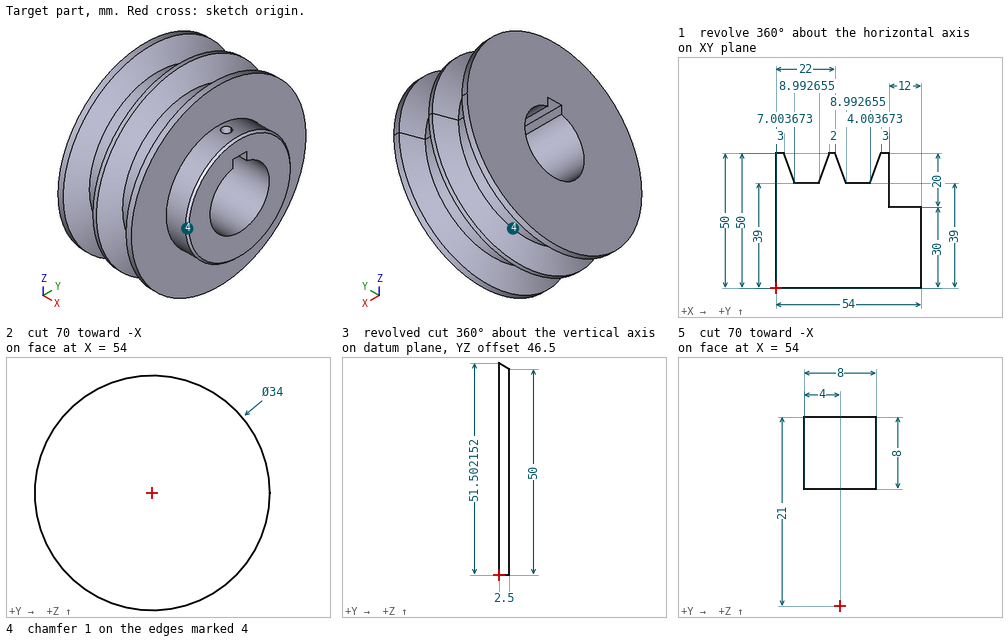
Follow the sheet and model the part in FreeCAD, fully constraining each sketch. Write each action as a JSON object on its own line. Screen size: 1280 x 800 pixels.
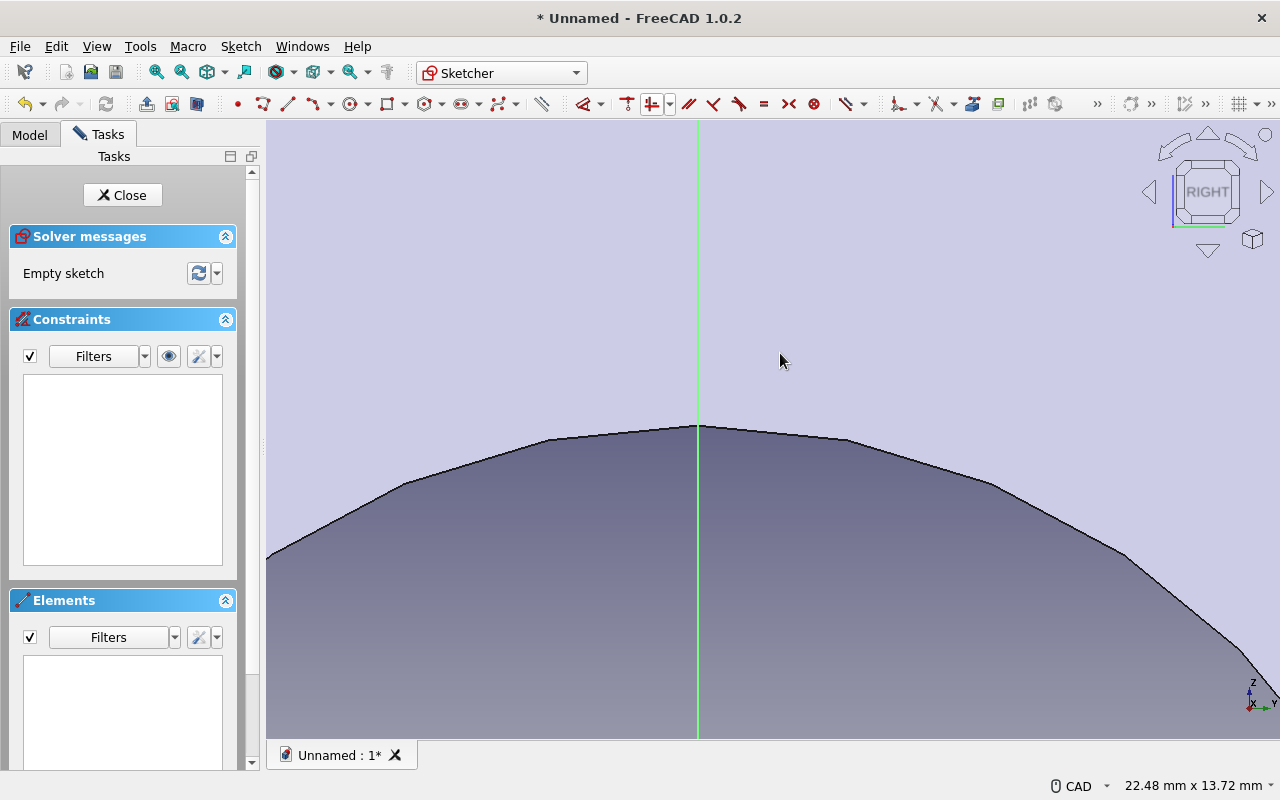
{"action": "key", "text": "g r"}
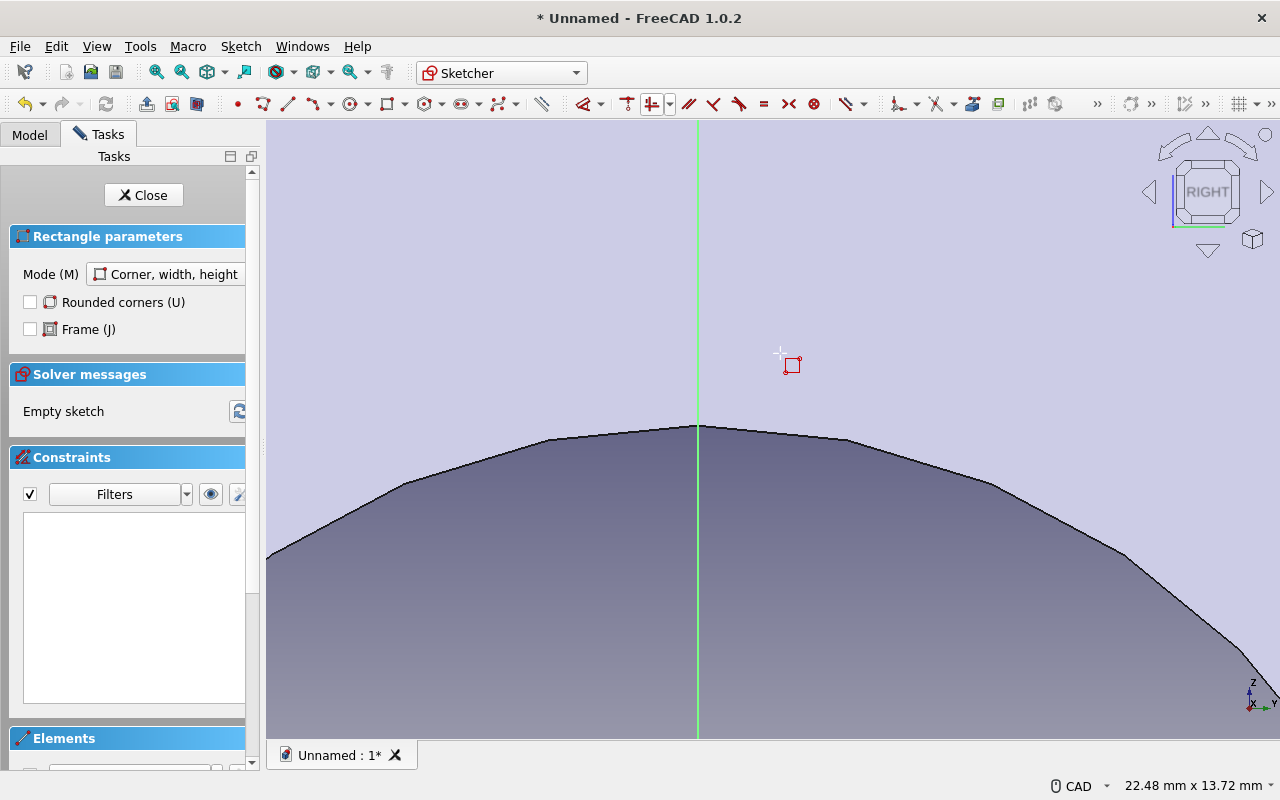
{"action": "left_click", "coordinate": [517, 245]}
{"action": "mouse_move", "coordinate": [878, 606]}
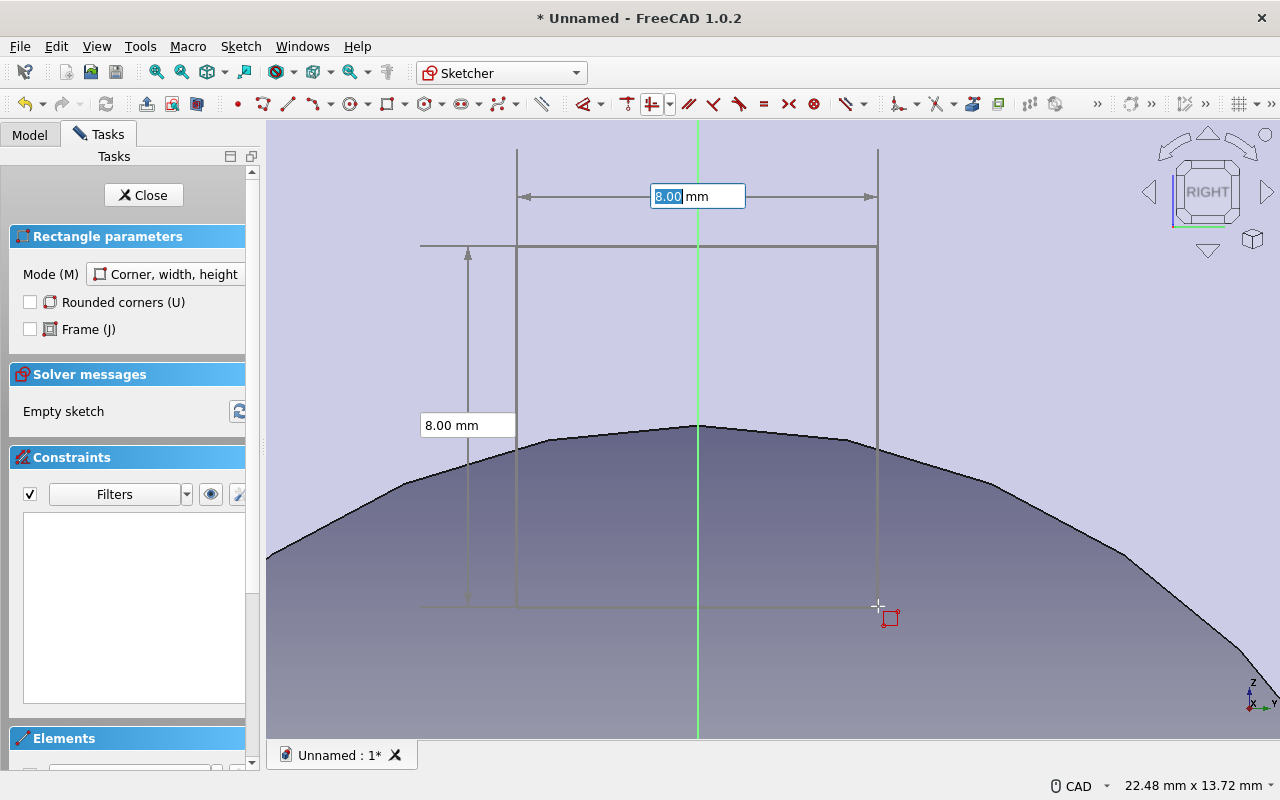
{"action": "type", "text": "8"}
{"action": "key", "text": "Tab"}
{"action": "type", "text": "8"}
{"action": "key", "text": "Return"}
{"action": "key", "text": "Escape"}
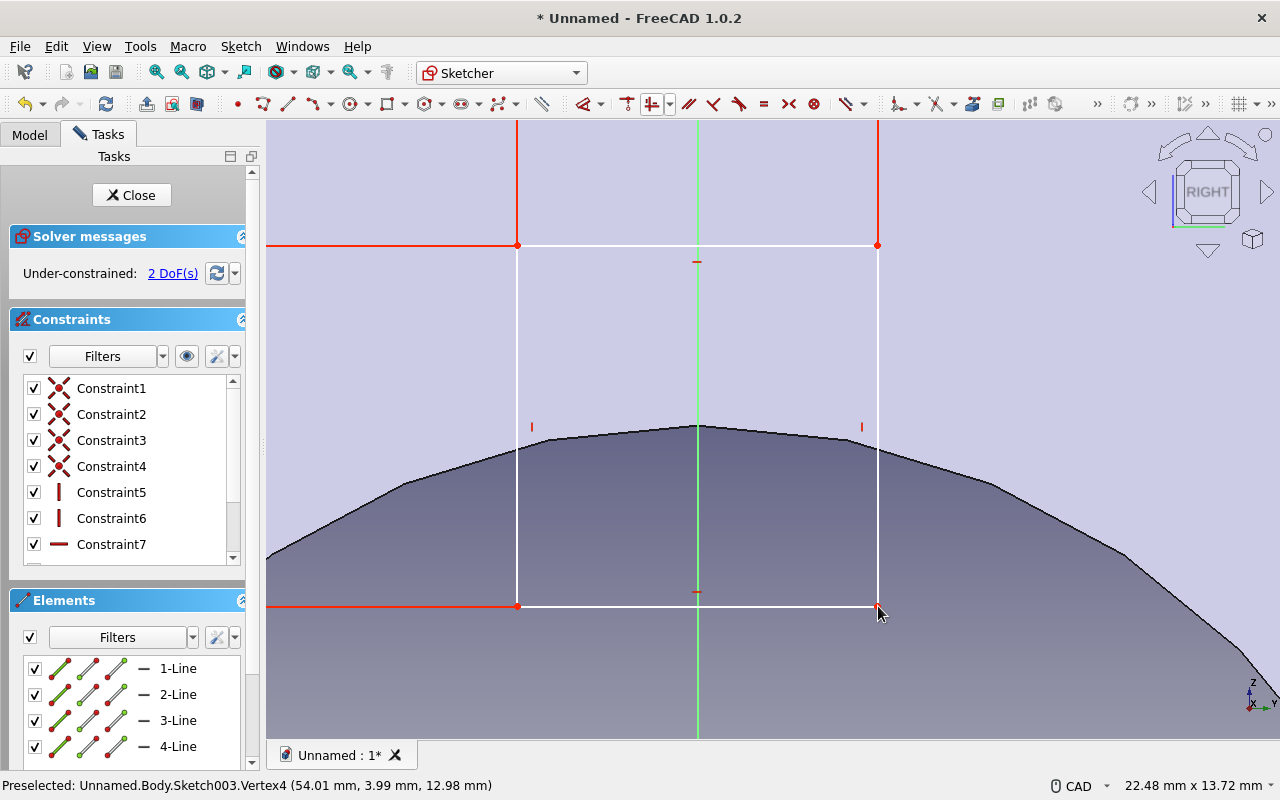
{"action": "key", "text": "d"}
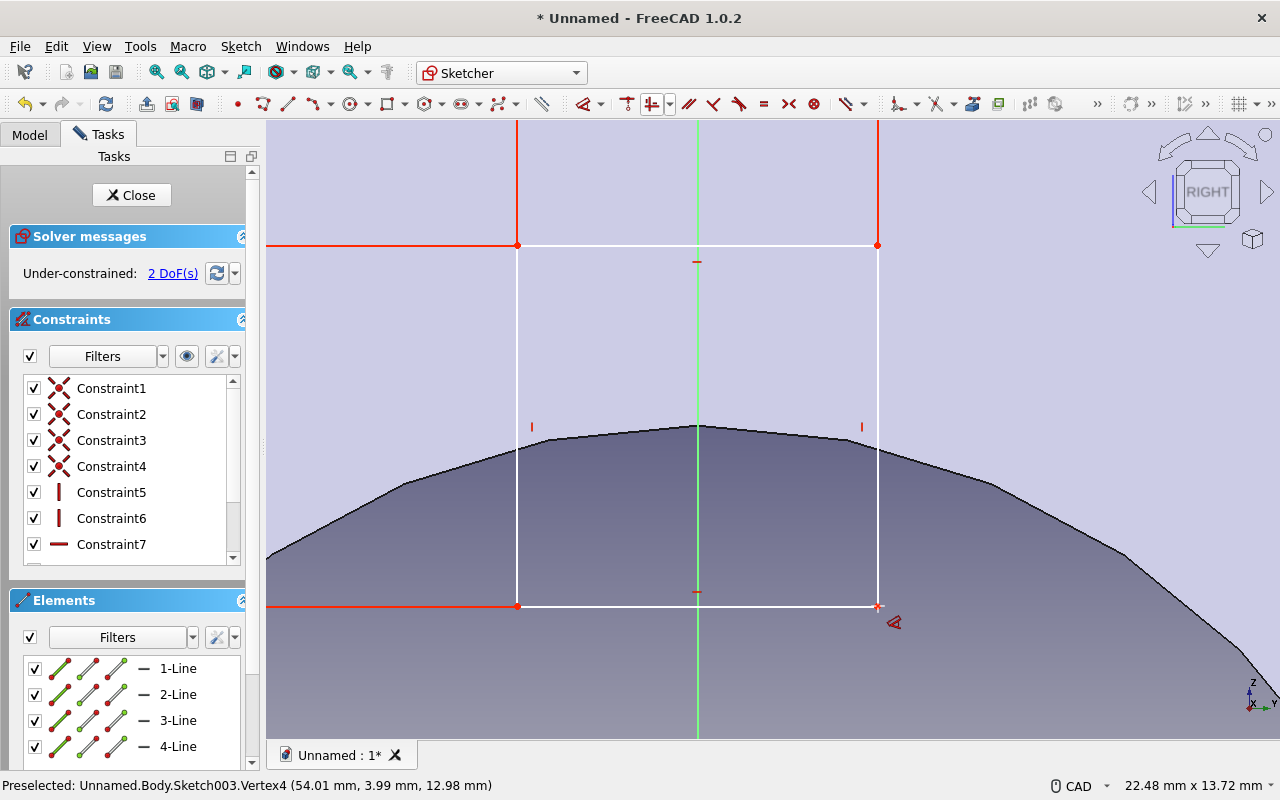
{"action": "left_click", "coordinate": [517, 246]}
{"action": "left_click", "coordinate": [607, 212]}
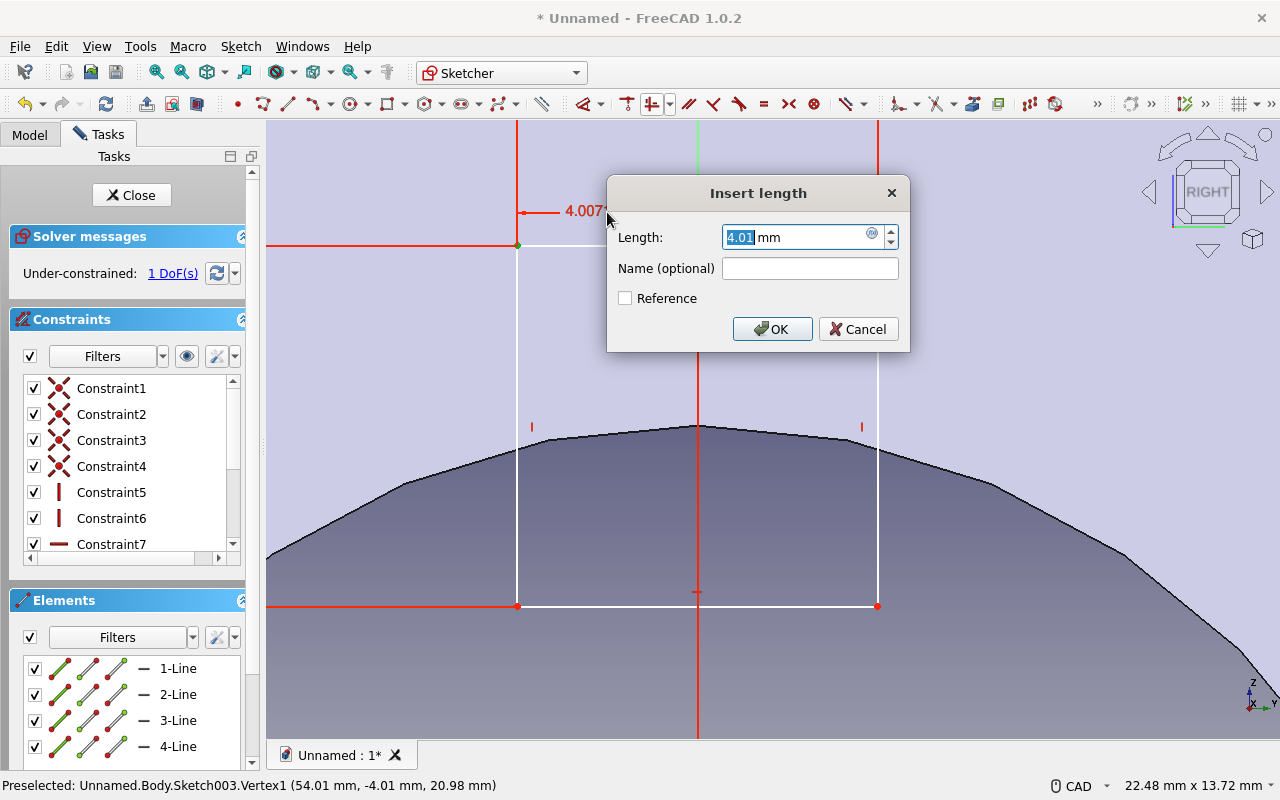
{"action": "type", "text": "4"}
{"action": "key", "text": "Return"}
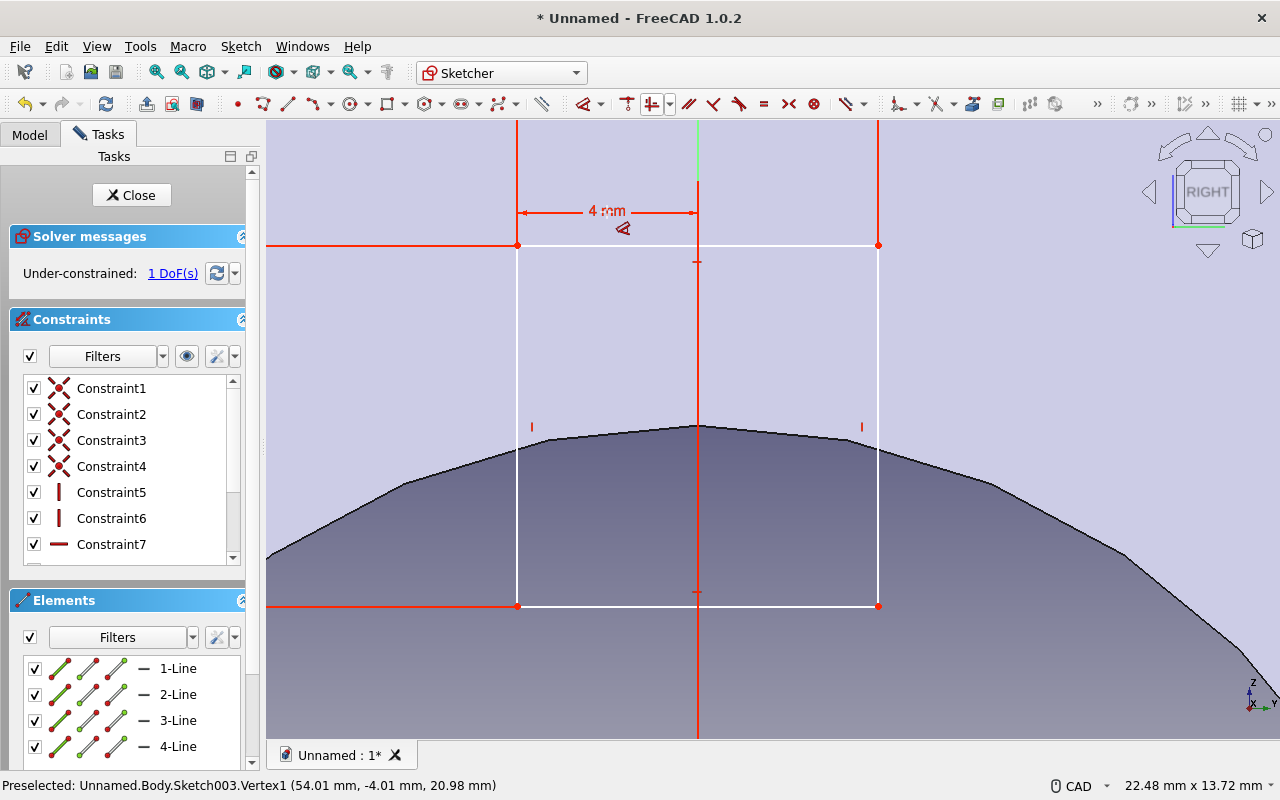
{"action": "left_click", "coordinate": [517, 246]}
{"action": "left_click", "coordinate": [483, 479]}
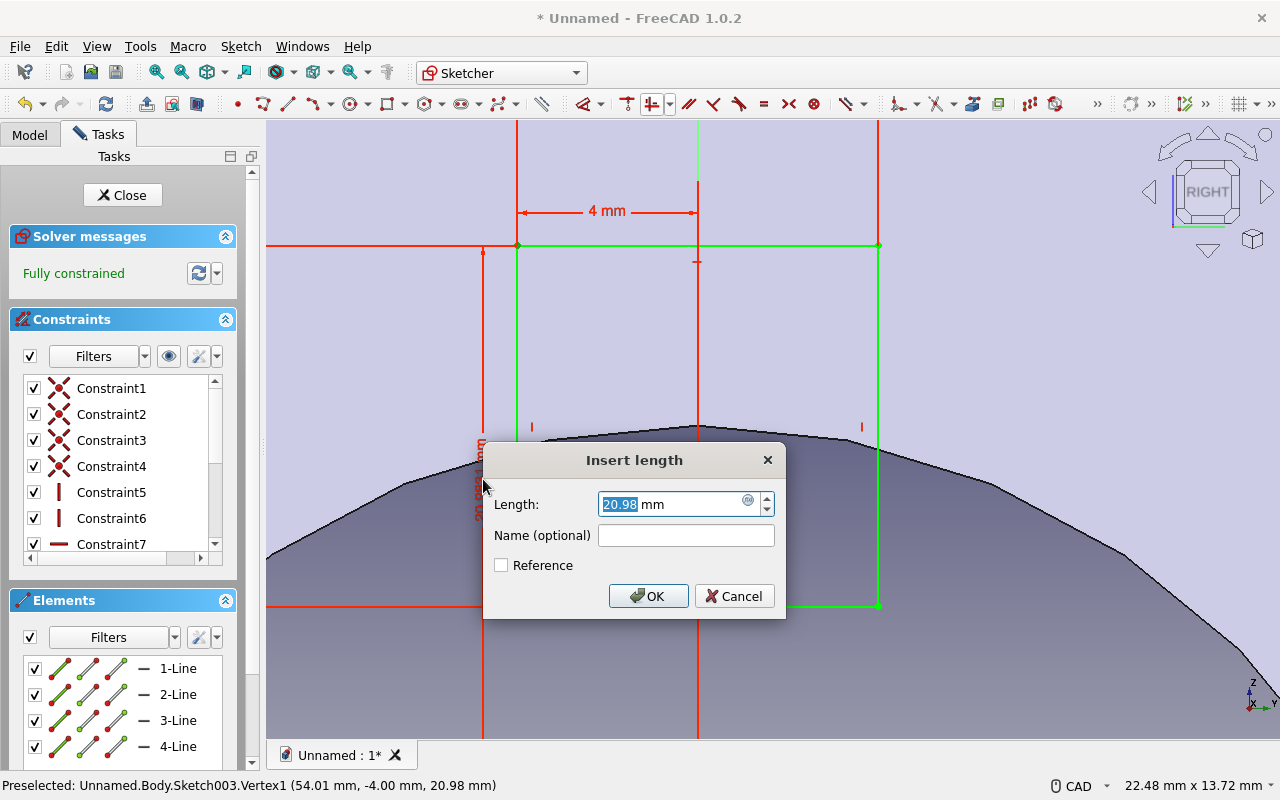
{"action": "type", "text": "21"}
{"action": "key", "text": "Return"}
{"action": "key", "text": "Escape"}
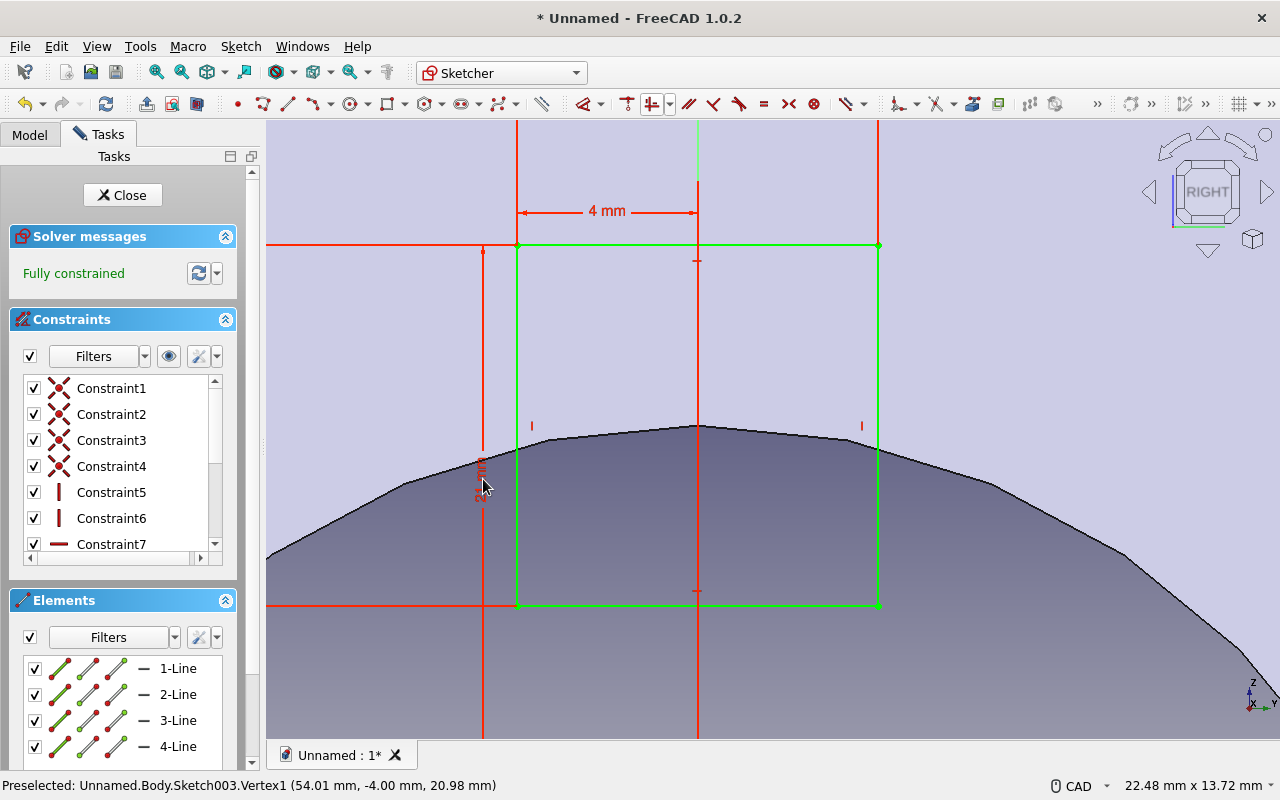
{"action": "left_click", "coordinate": [123, 195]}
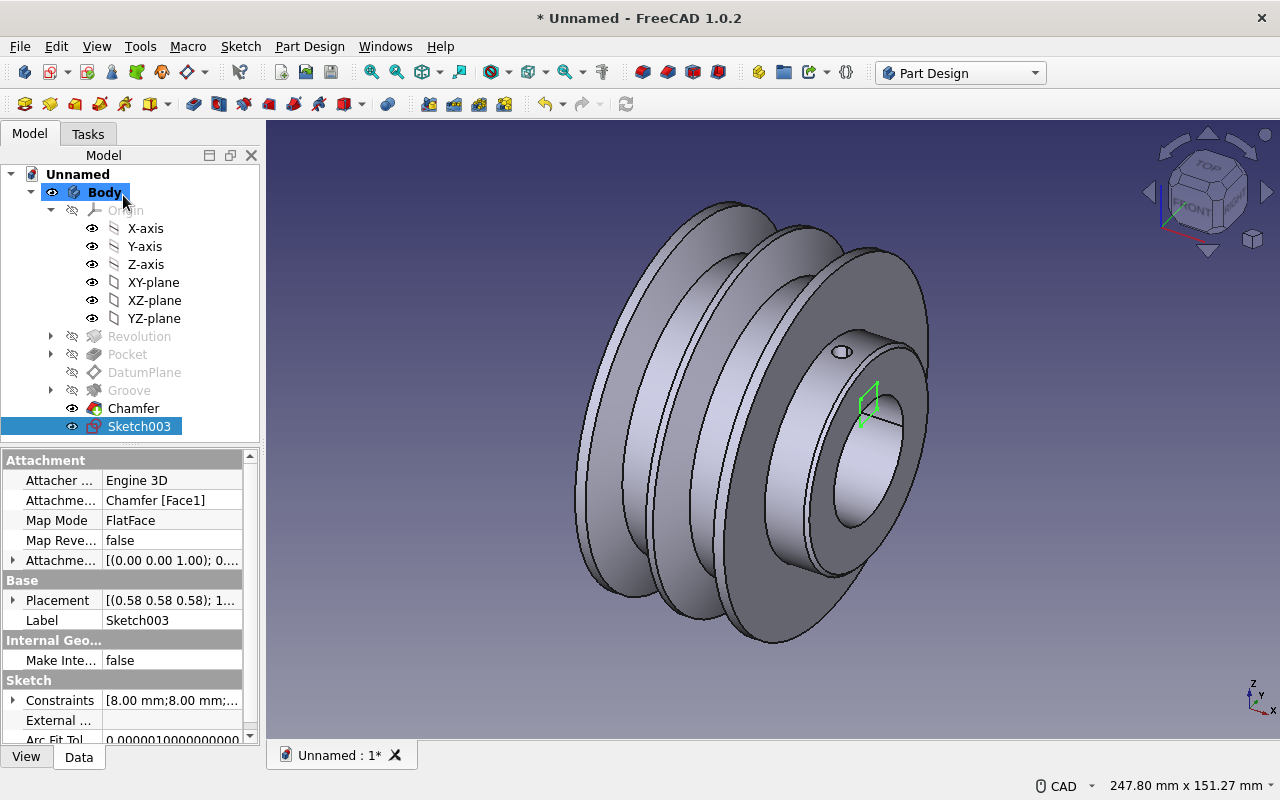
{"action": "left_click", "coordinate": [194, 104]}